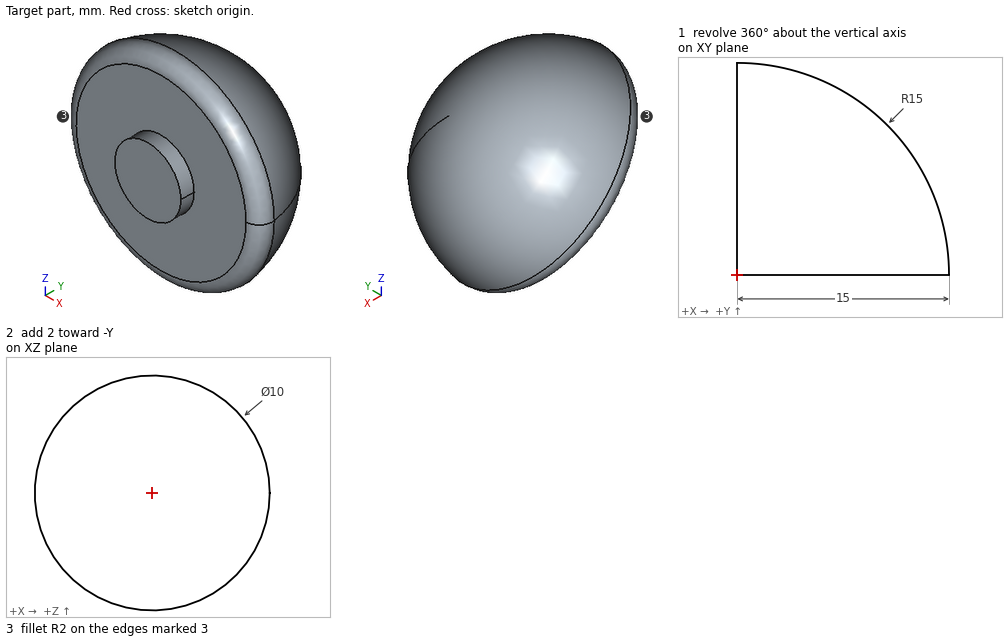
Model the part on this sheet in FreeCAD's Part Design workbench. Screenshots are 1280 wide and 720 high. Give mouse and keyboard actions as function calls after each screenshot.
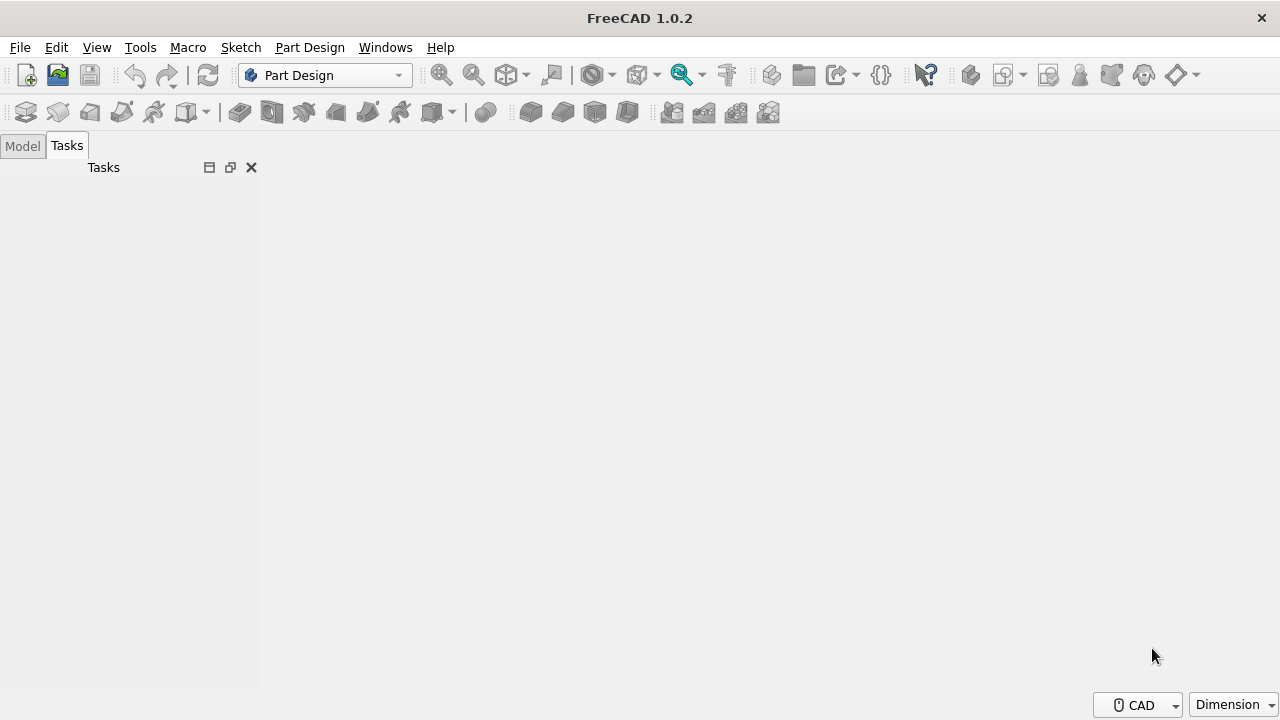
key(ctrl+n)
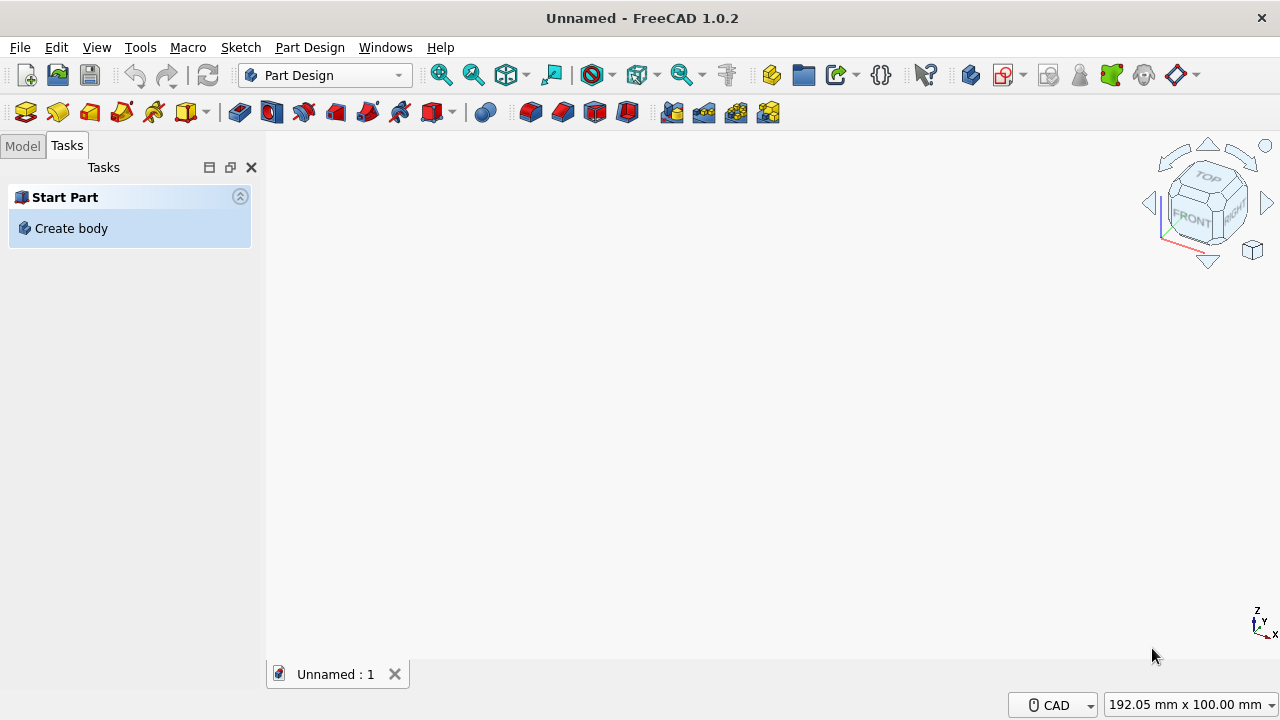
click(1004, 76)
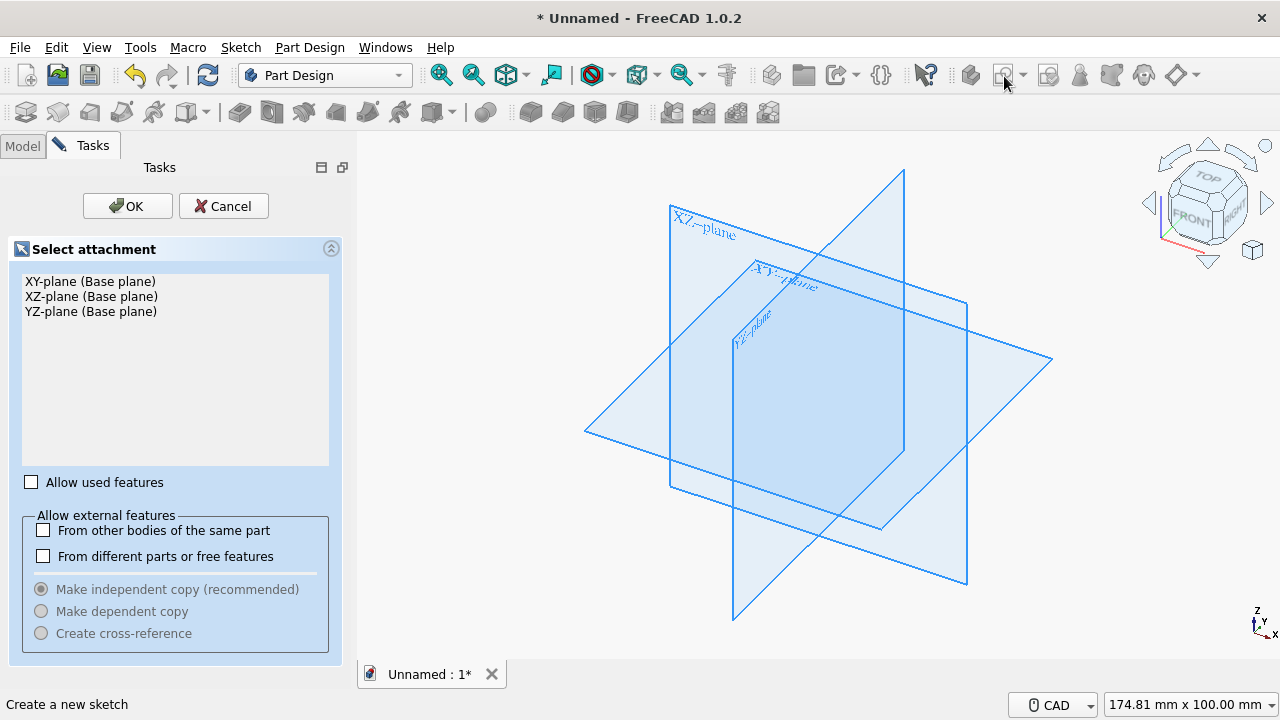
click(82, 282)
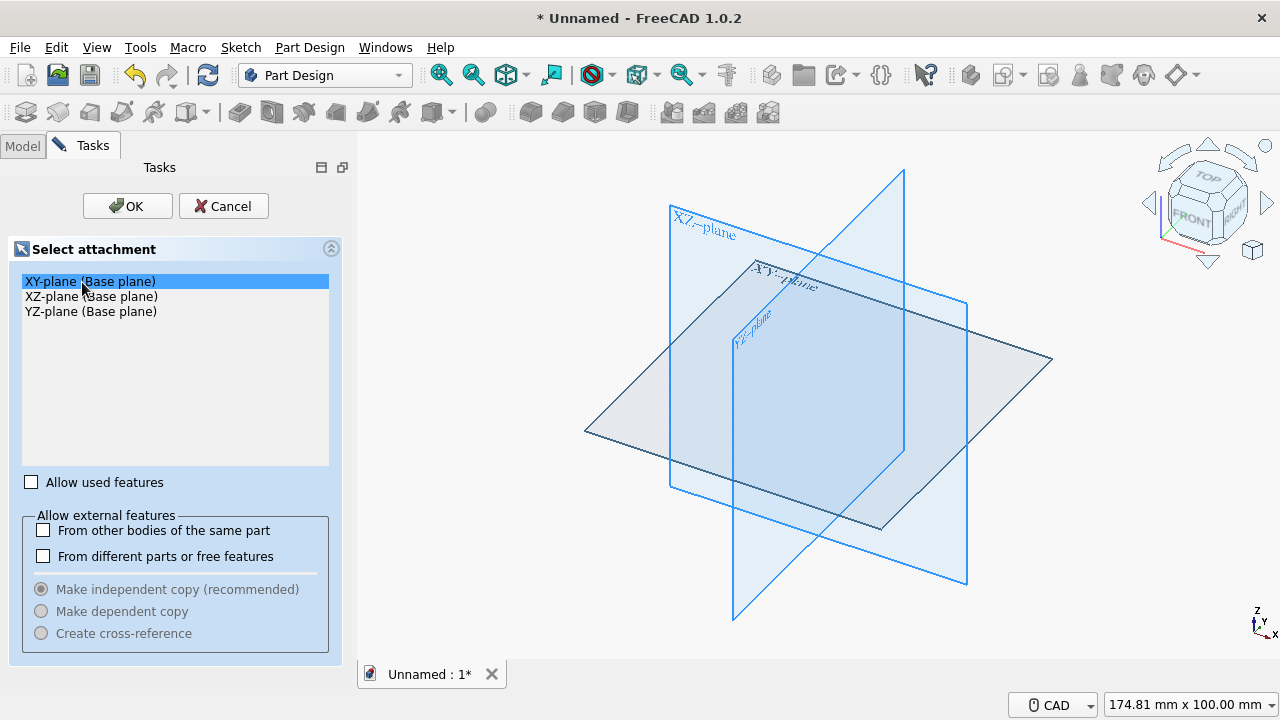
click(128, 206)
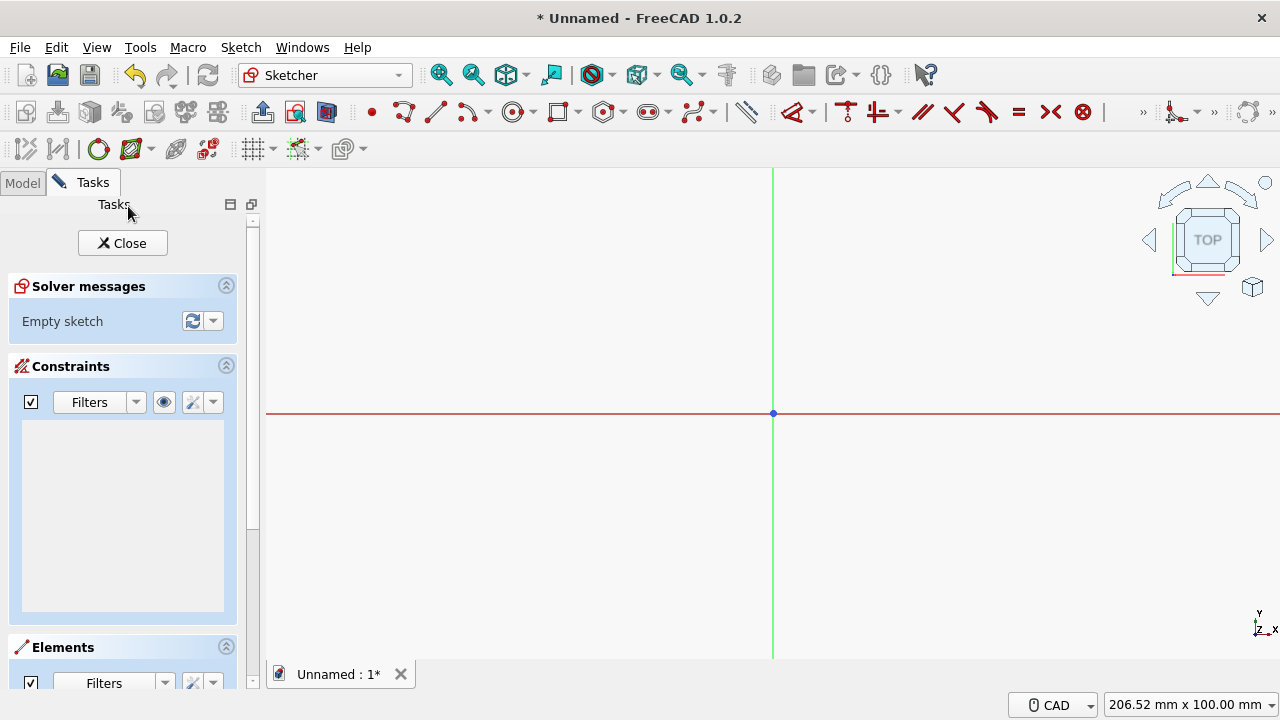
scroll(844, 365, up, 7)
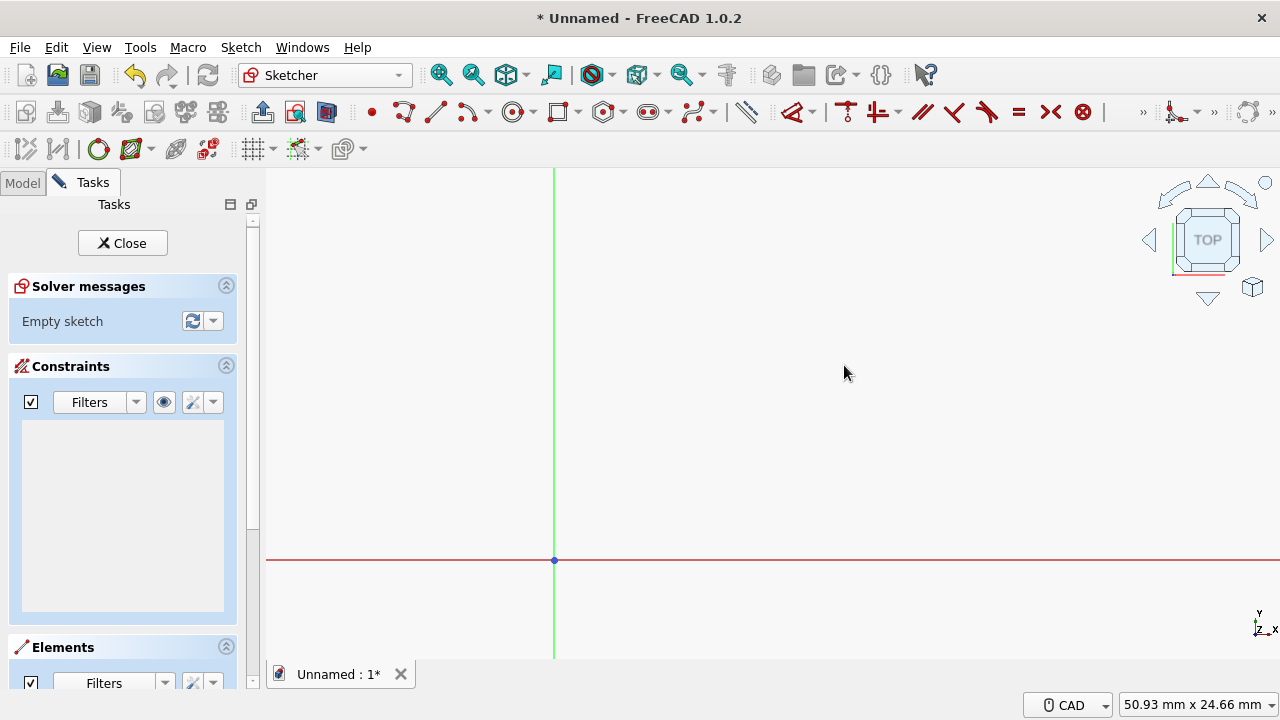
key(g)
key(m)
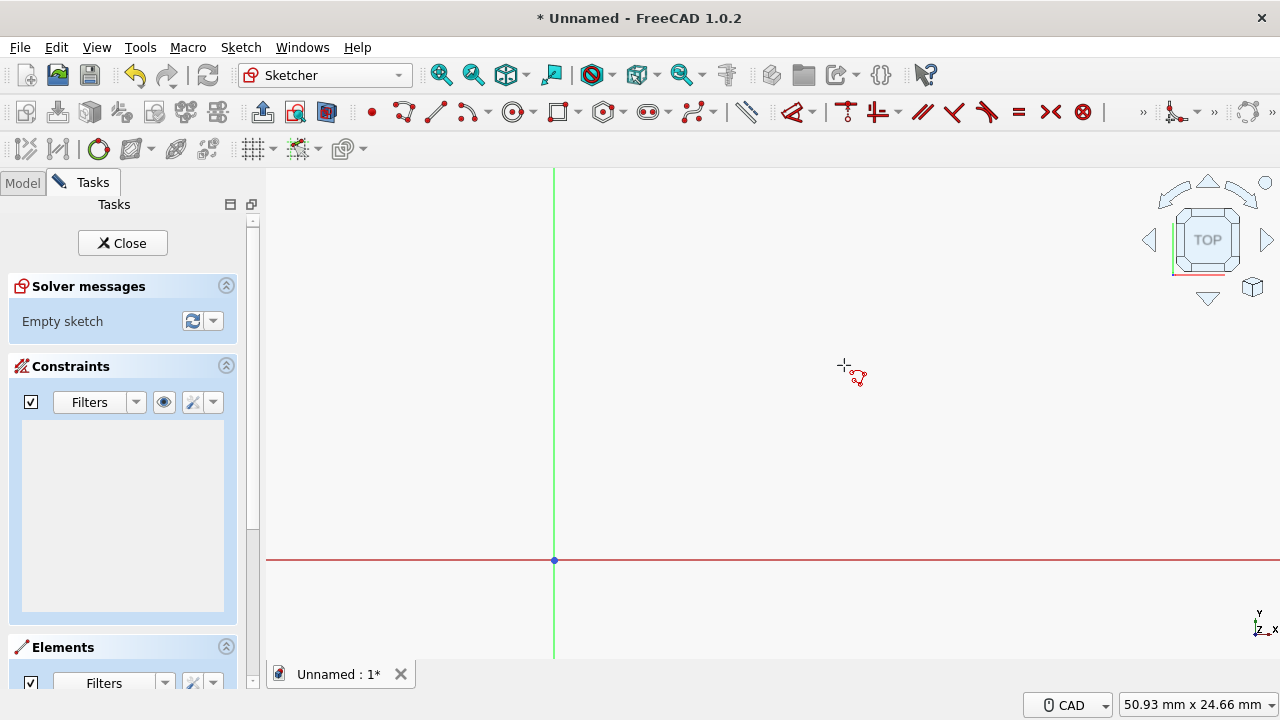
click(554, 262)
click(554, 560)
click(853, 551)
right_click(853, 551)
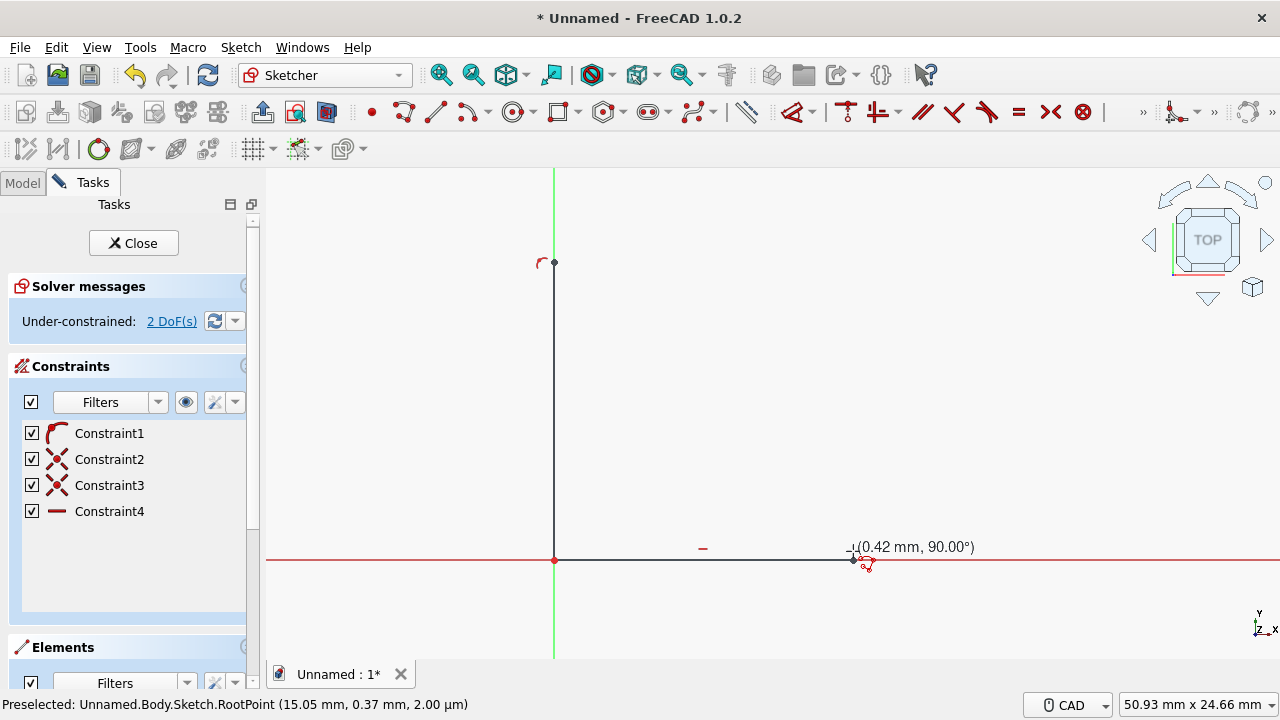
key(g)
key(3)
key(a)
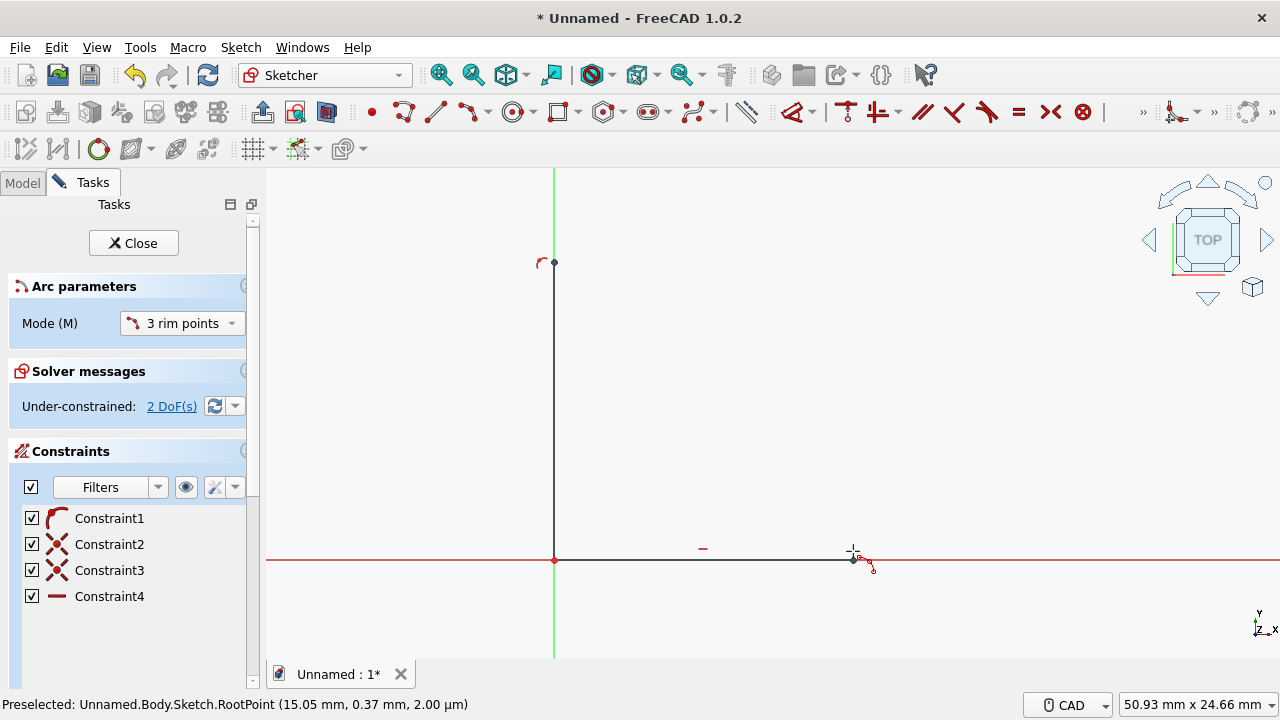
click(853, 551)
click(554, 263)
click(766, 349)
key(Escape)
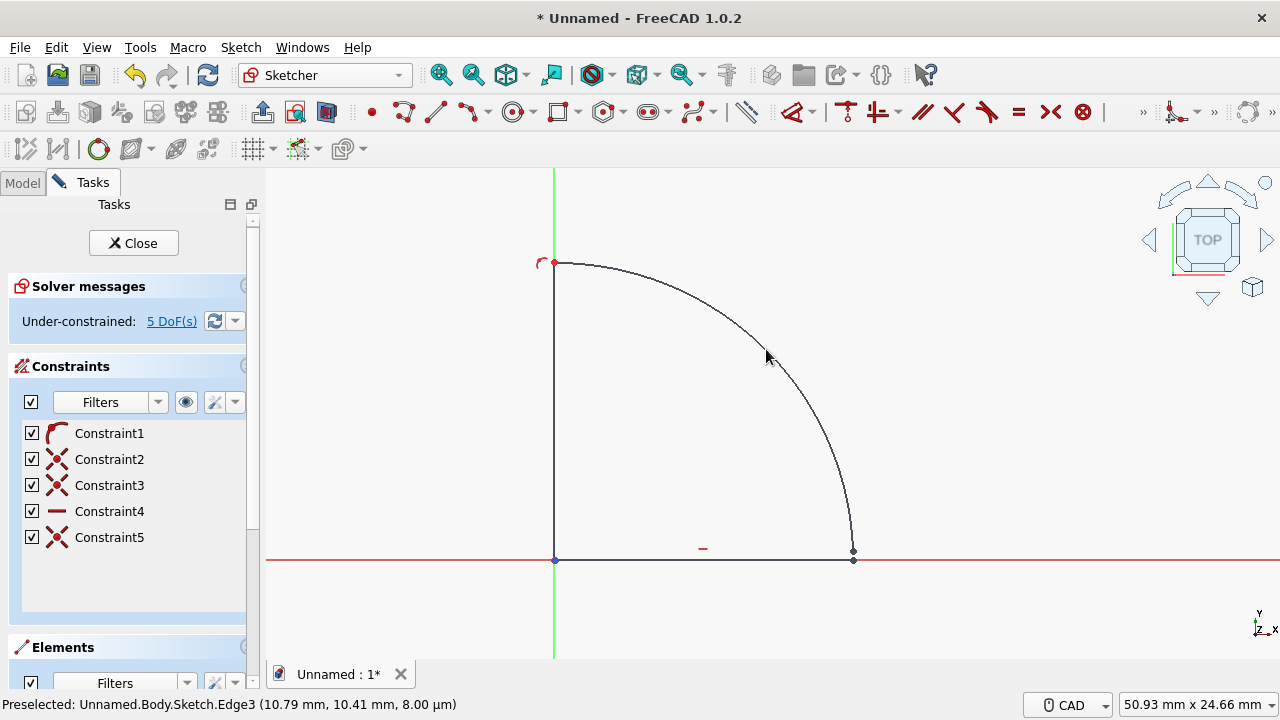
scroll(555, 560, up, 20)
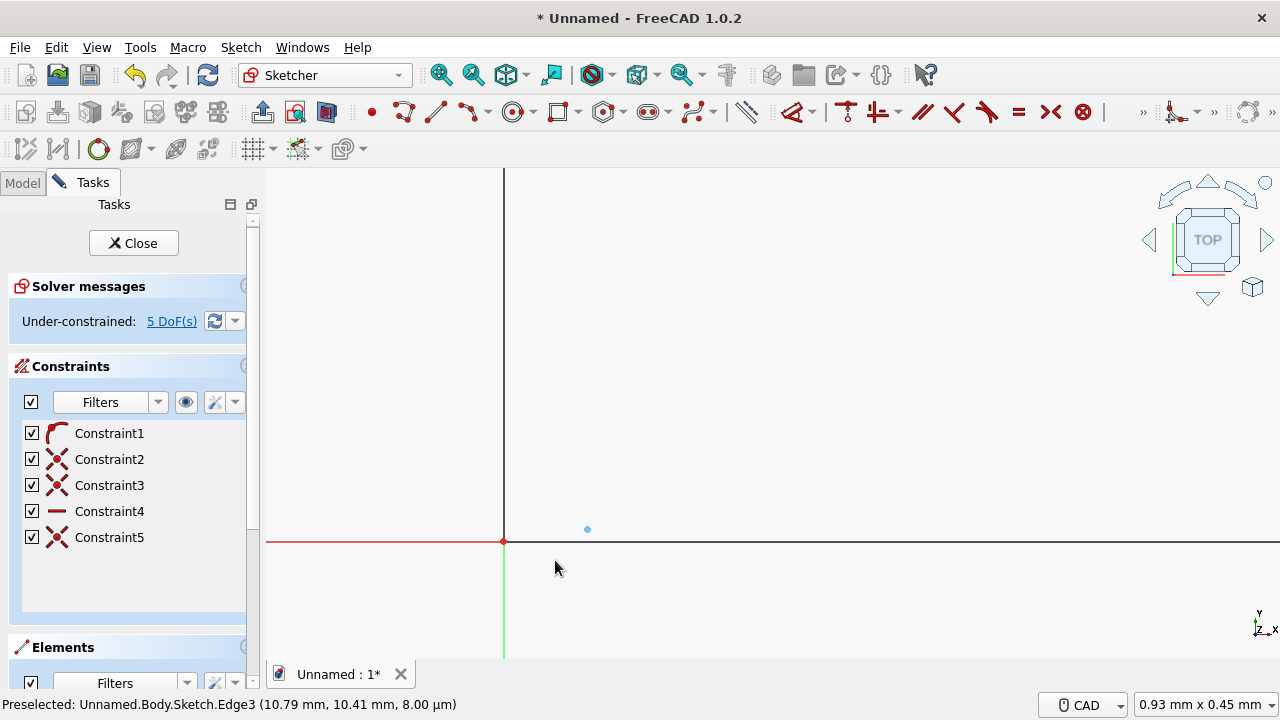
drag(494, 520, 598, 552)